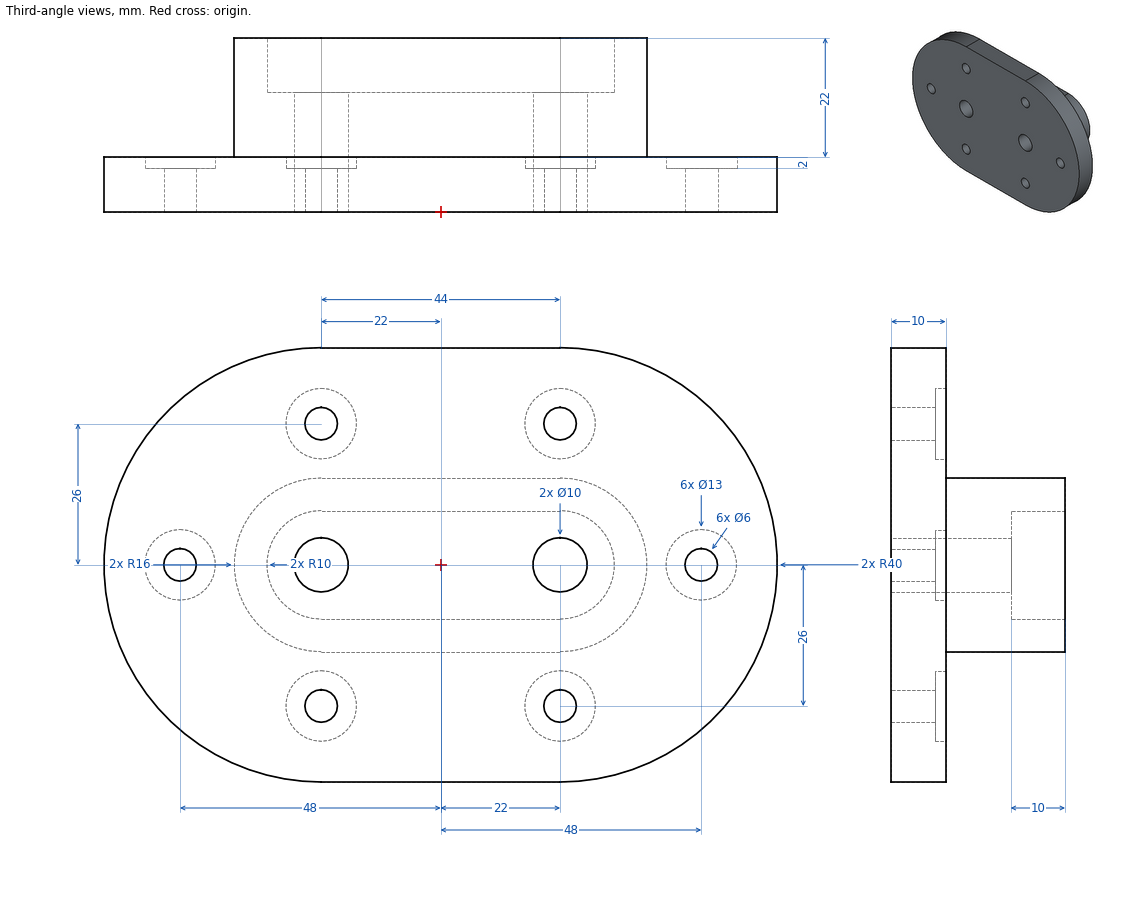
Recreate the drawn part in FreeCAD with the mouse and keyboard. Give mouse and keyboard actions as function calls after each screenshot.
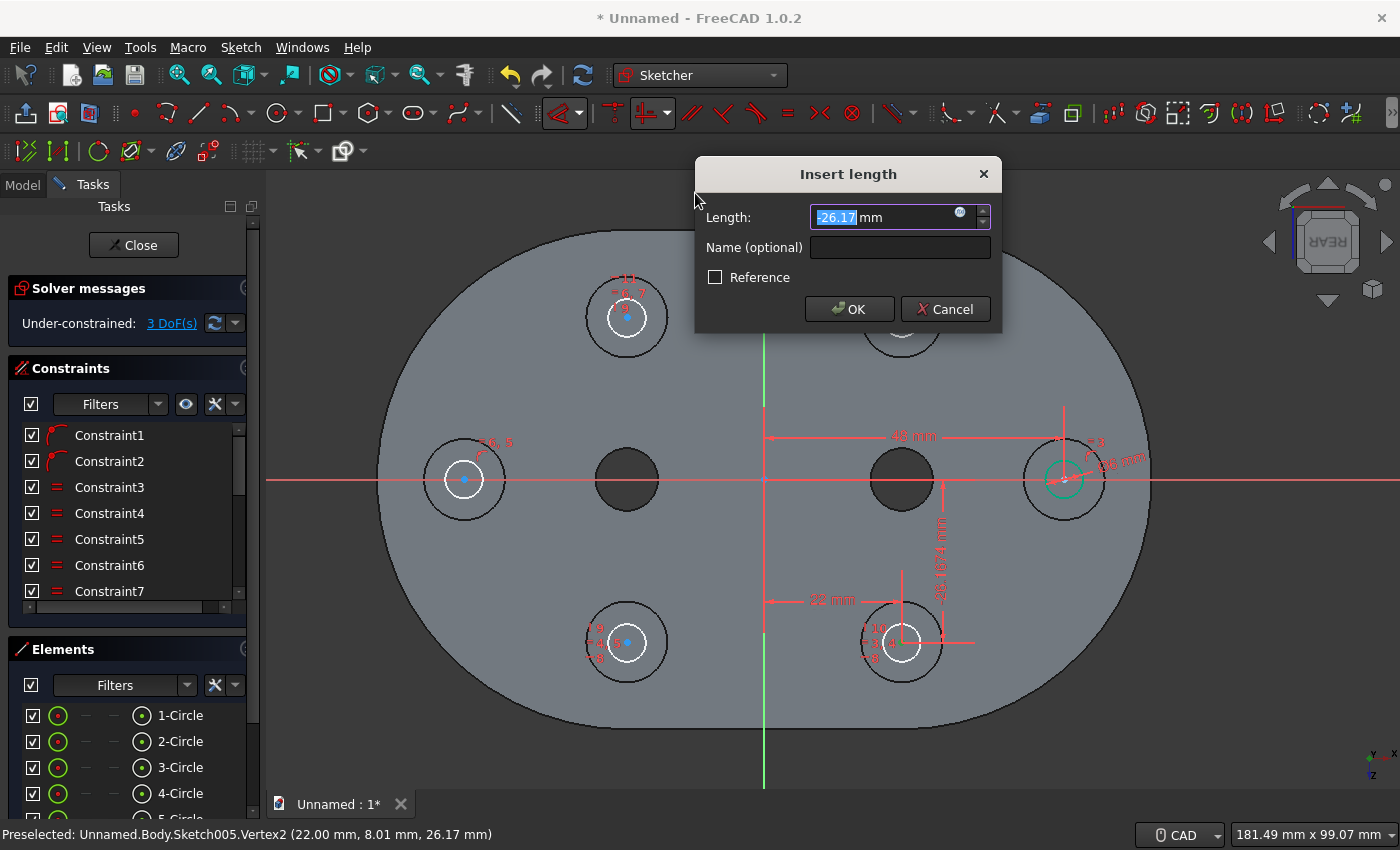
text(-26)
key(Return)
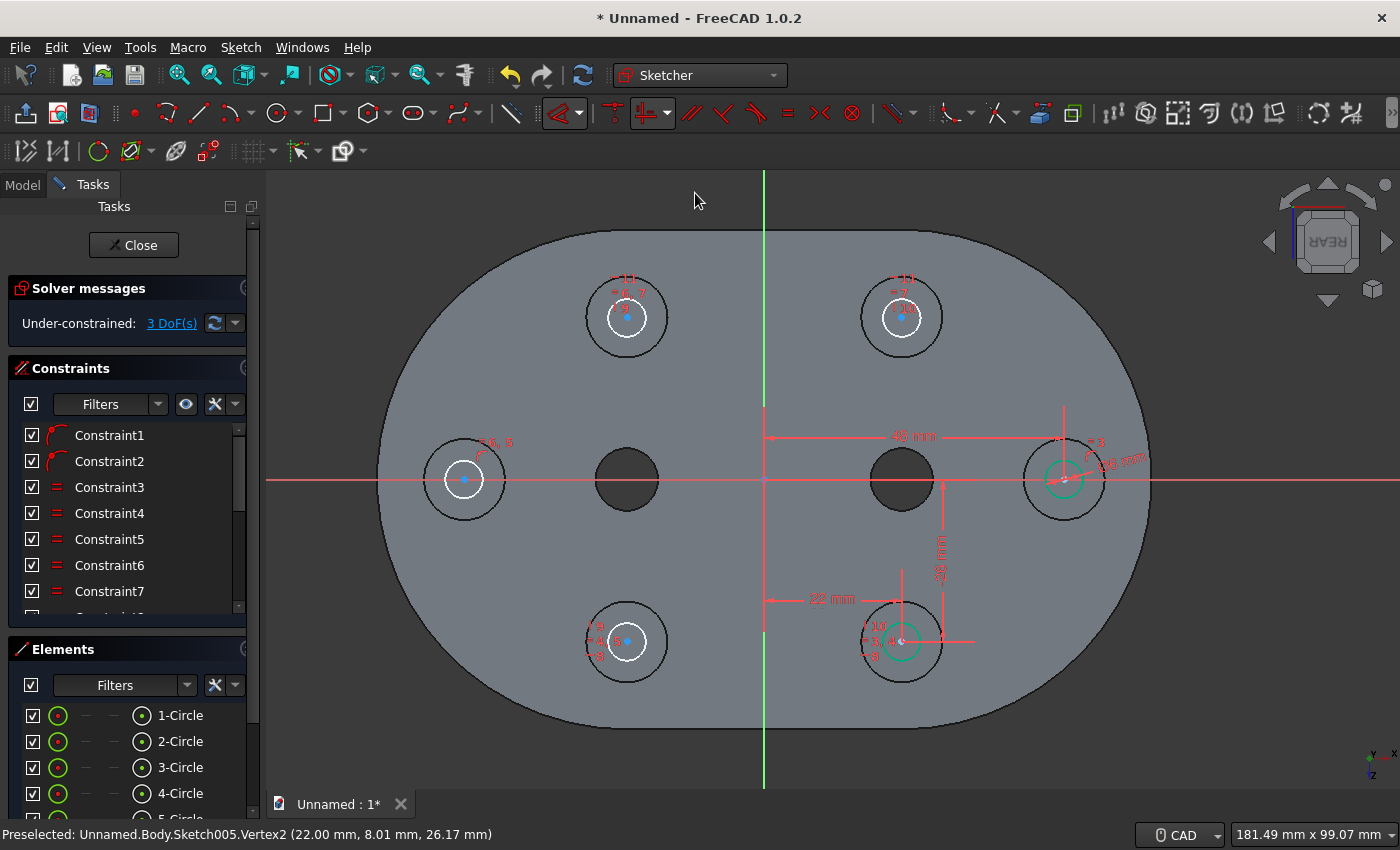
click(627, 642)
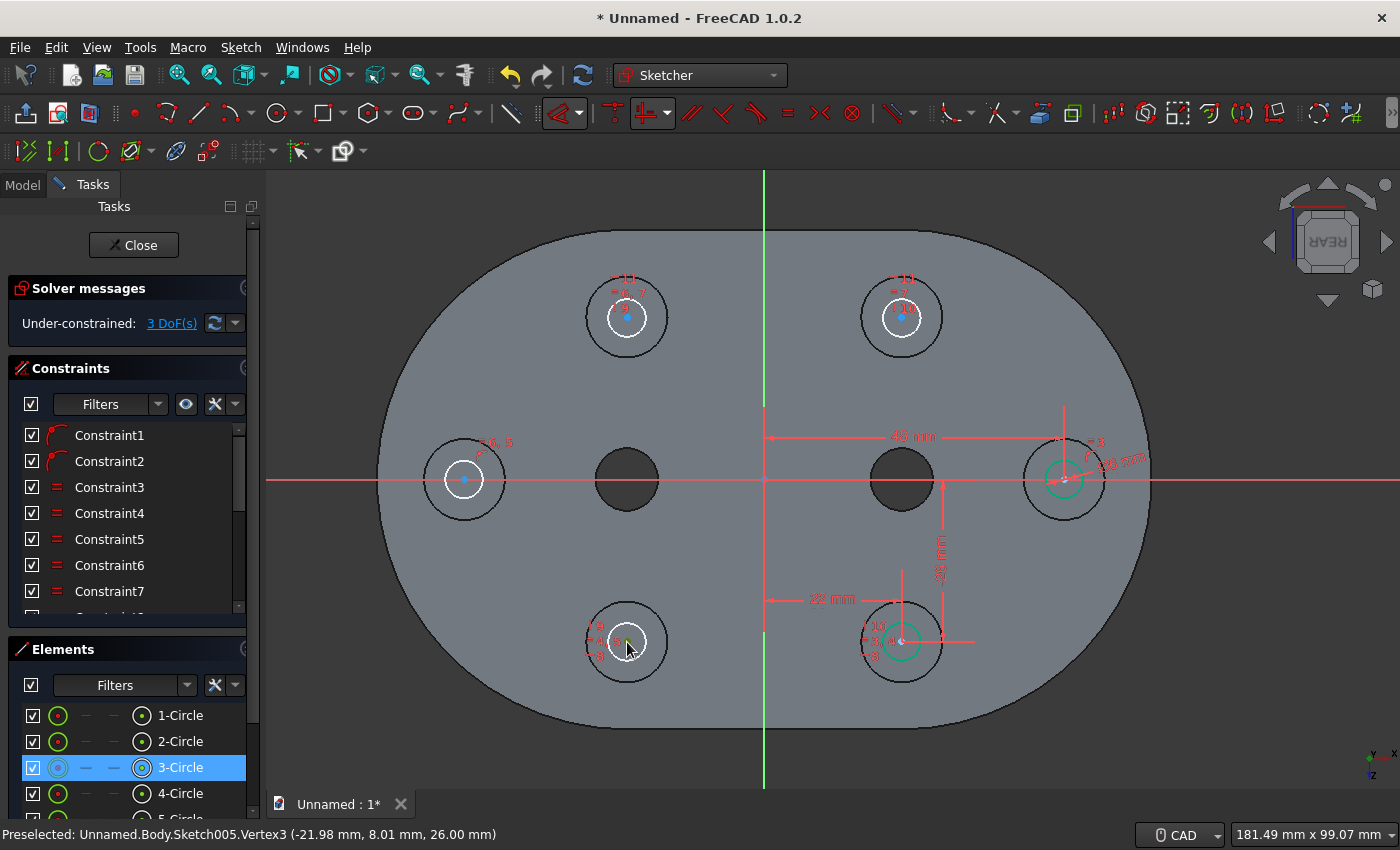
key(l)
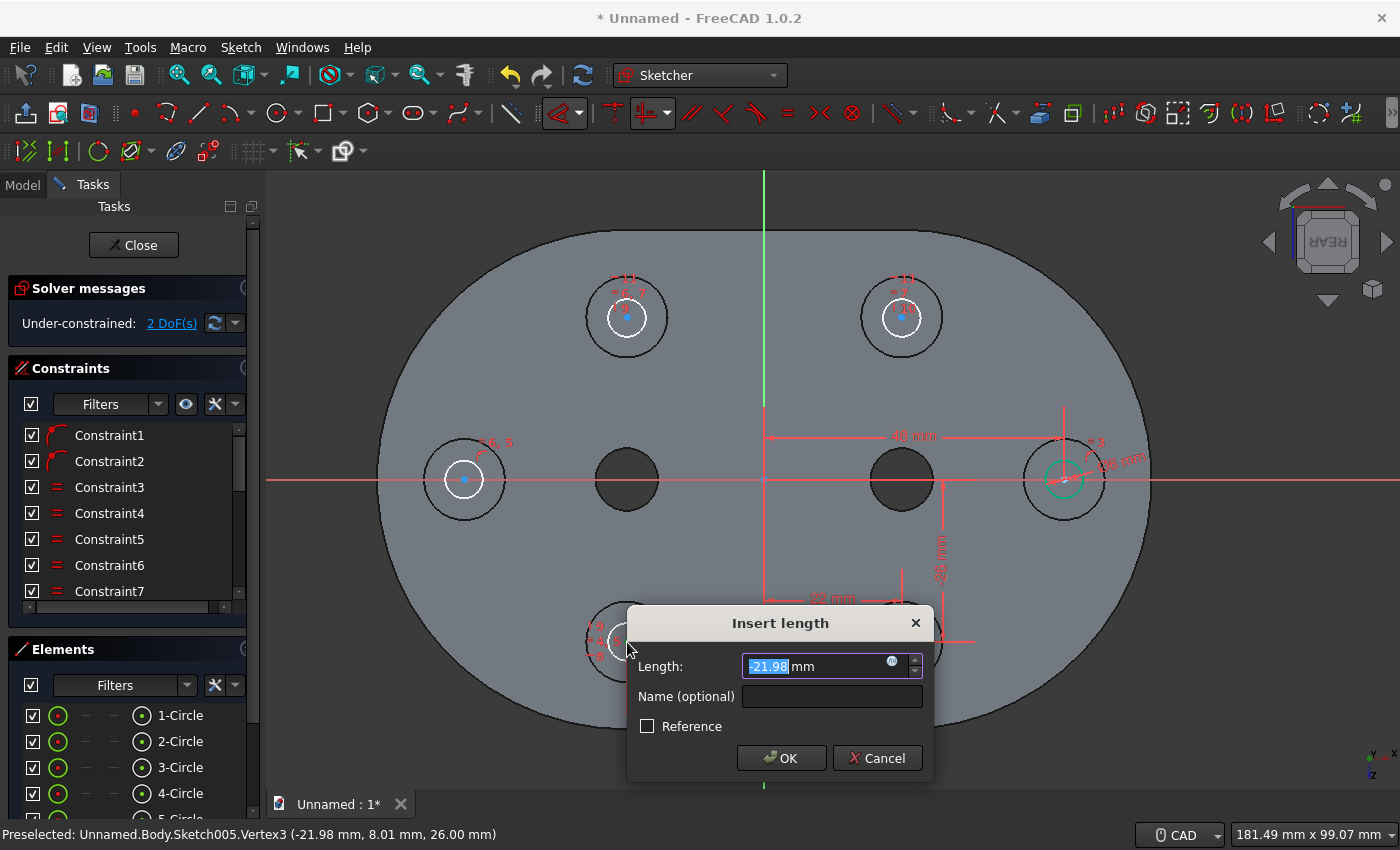
text(-22)
key(Return)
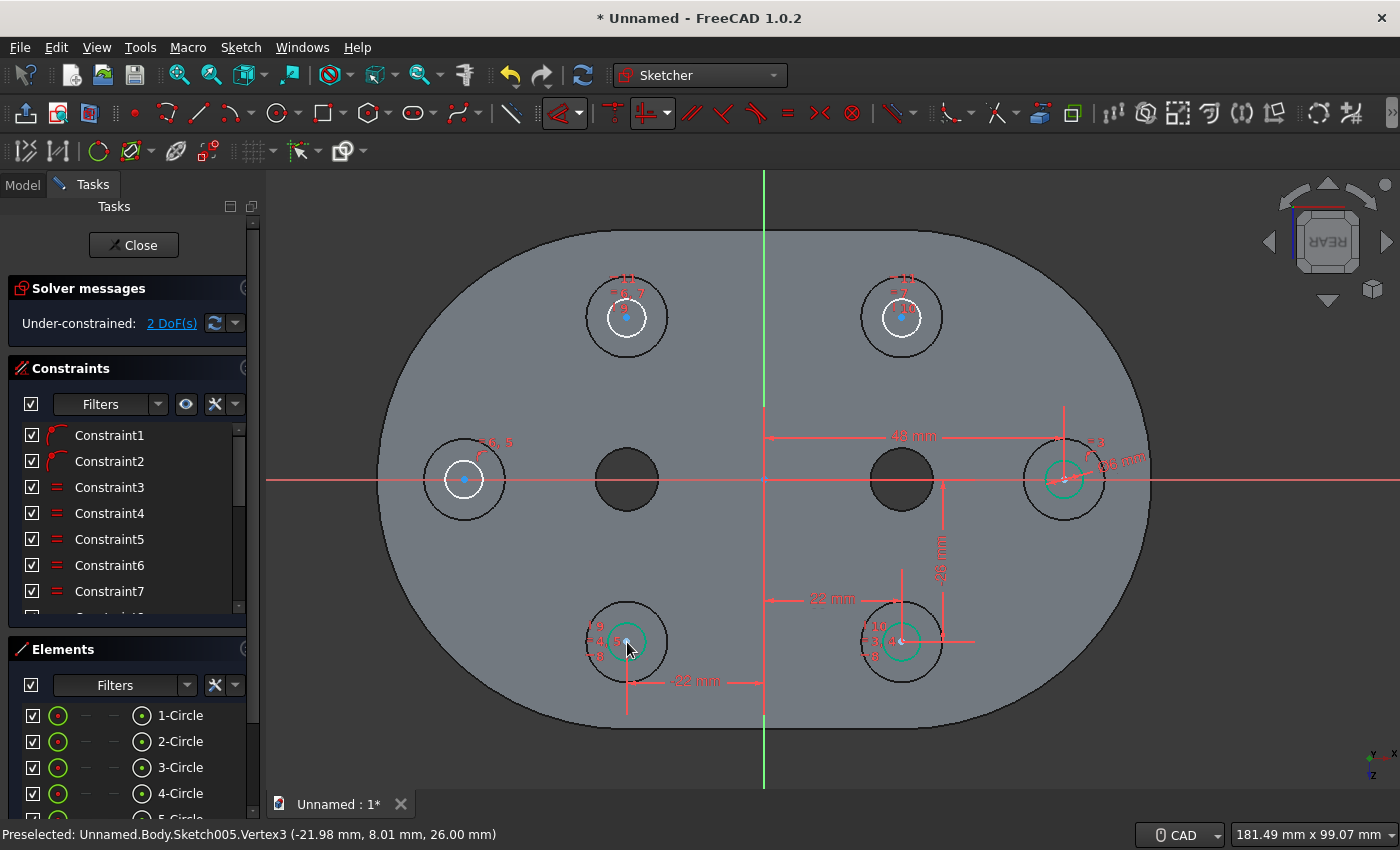
click(464, 479)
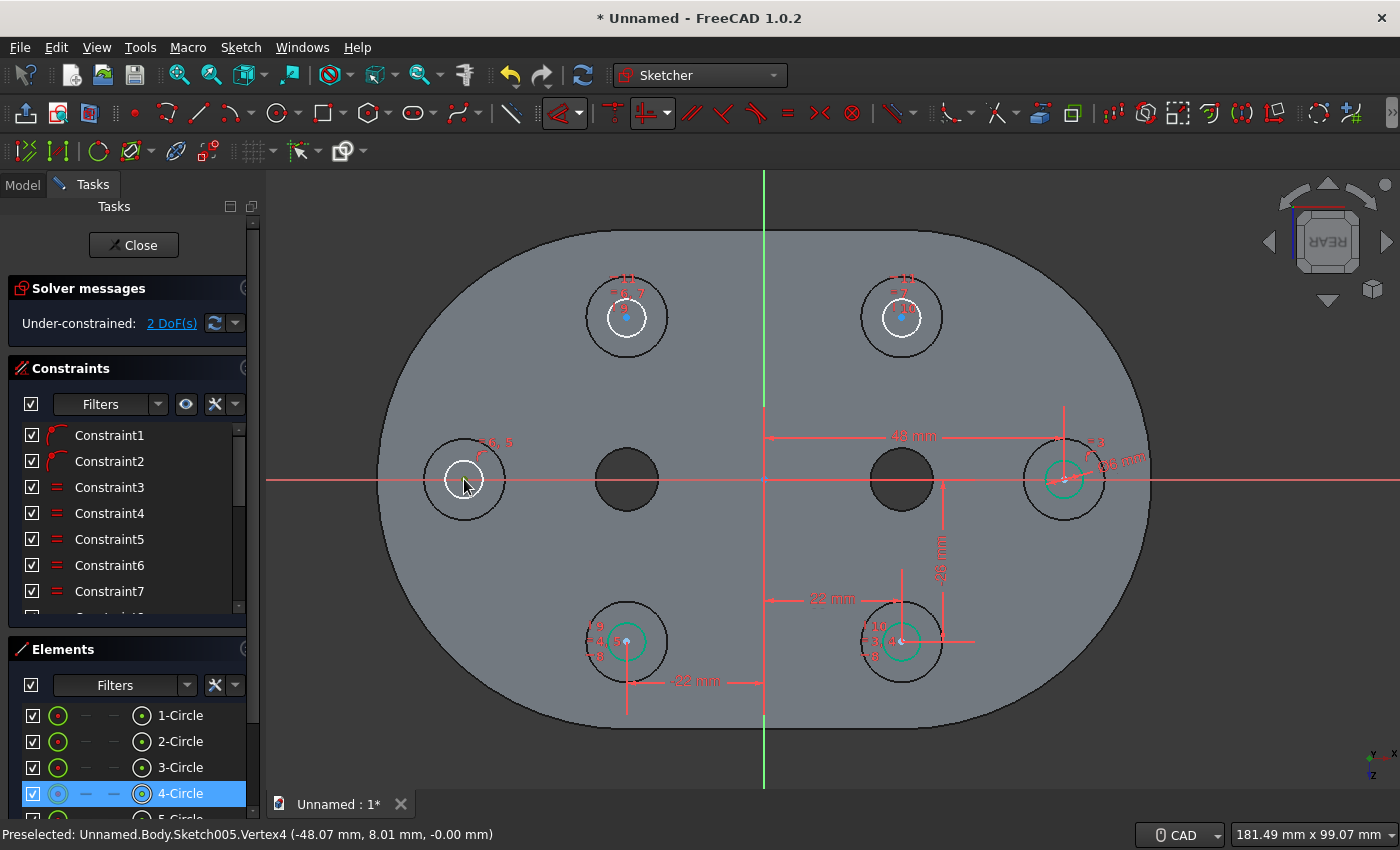
key(l)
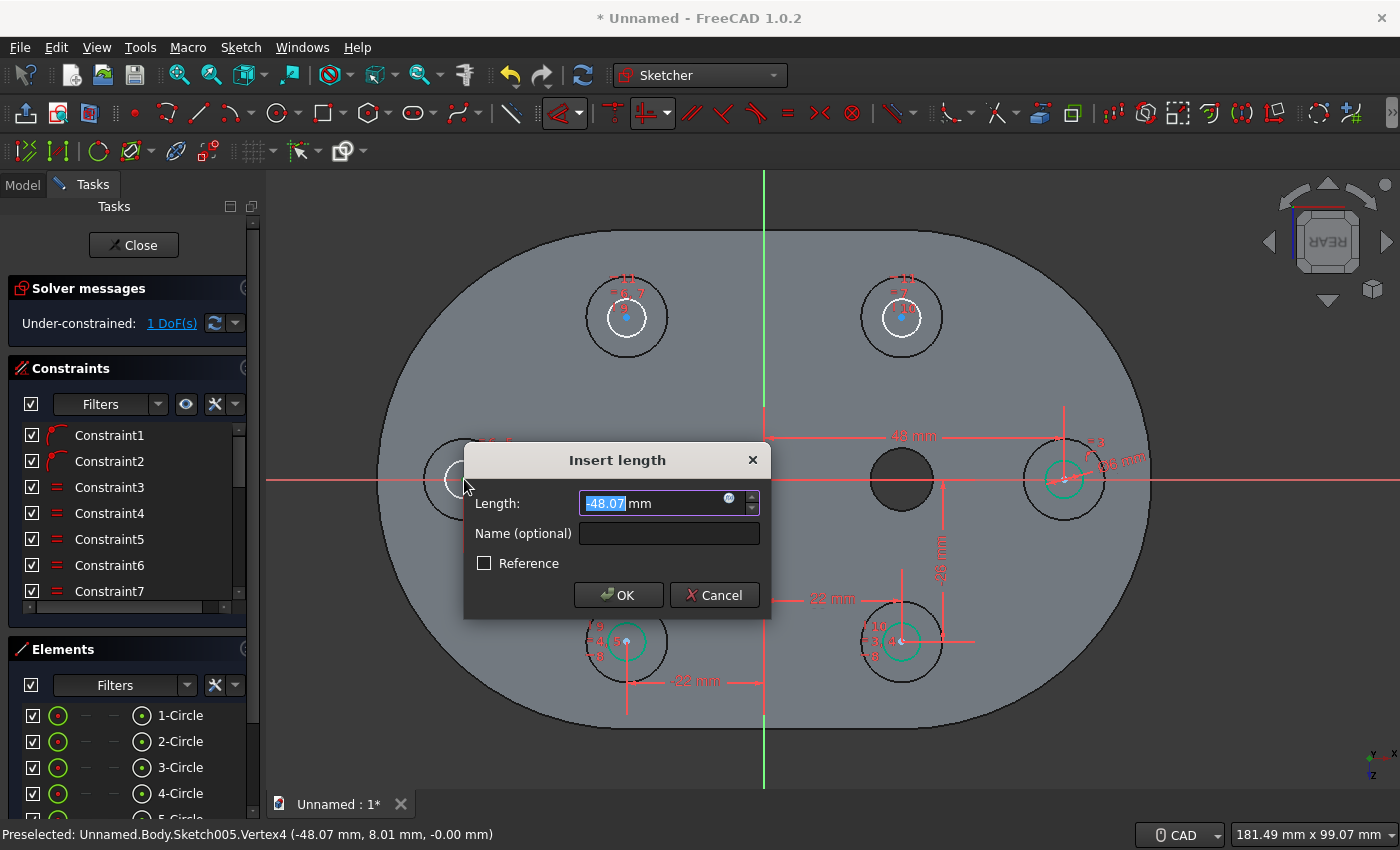
text(-48)
key(Return)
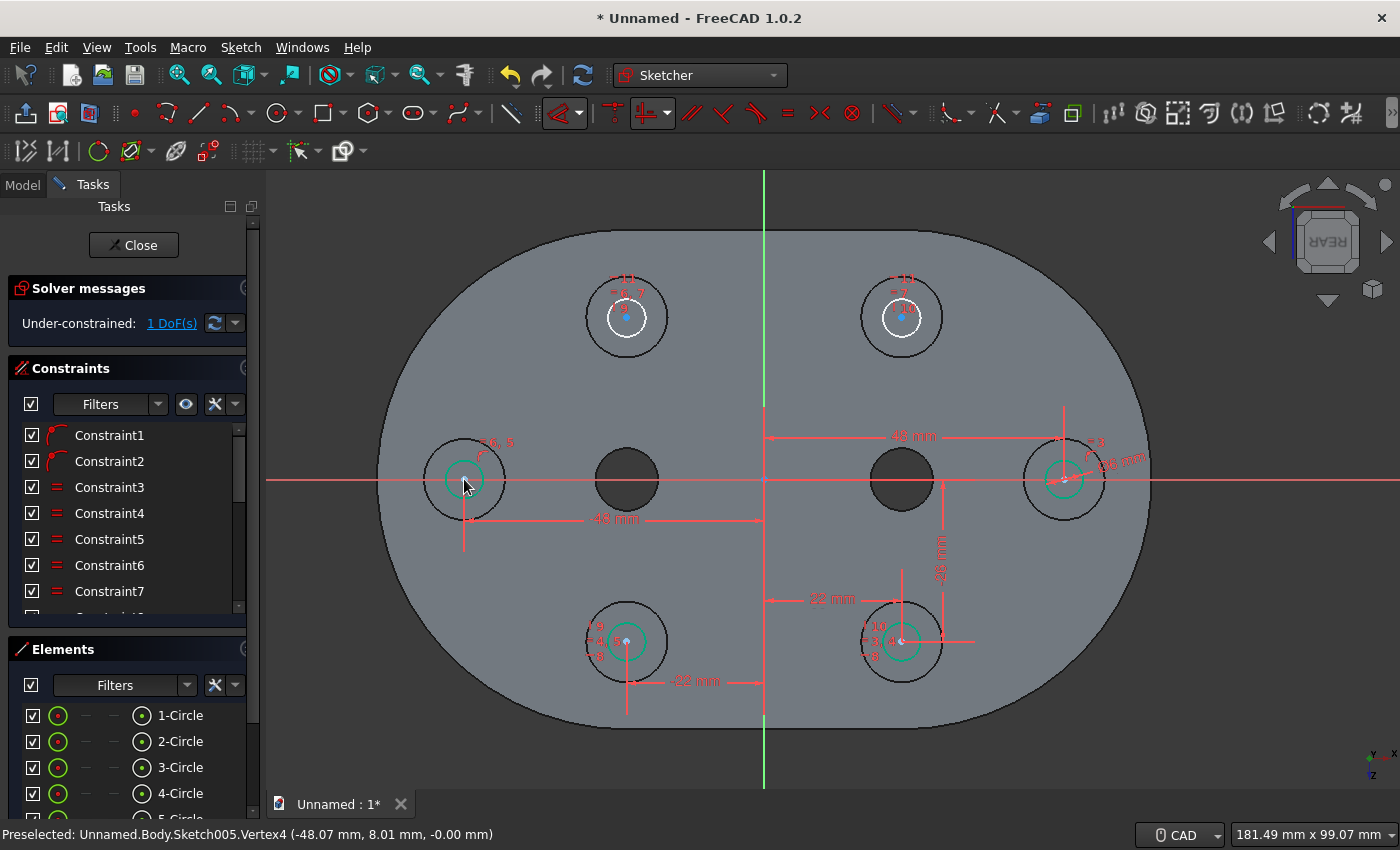
click(627, 318)